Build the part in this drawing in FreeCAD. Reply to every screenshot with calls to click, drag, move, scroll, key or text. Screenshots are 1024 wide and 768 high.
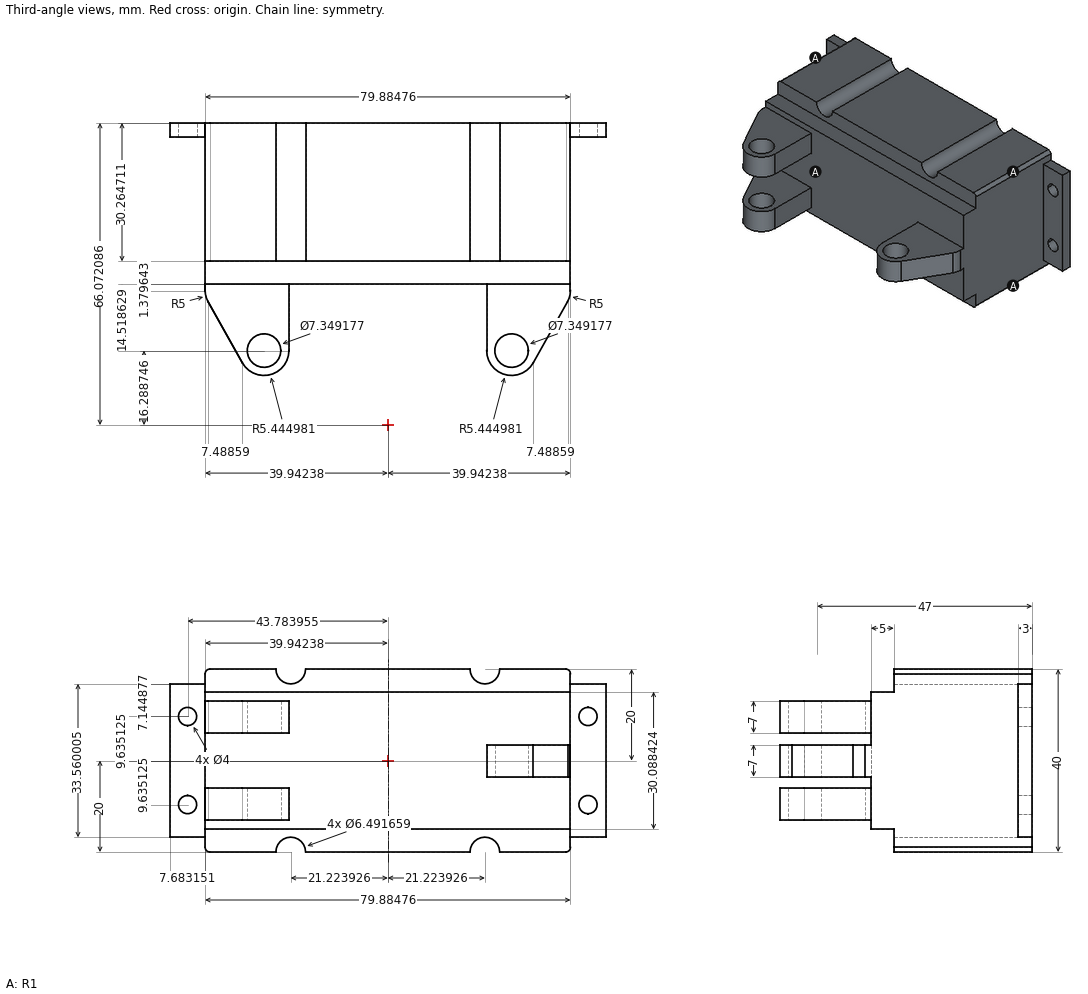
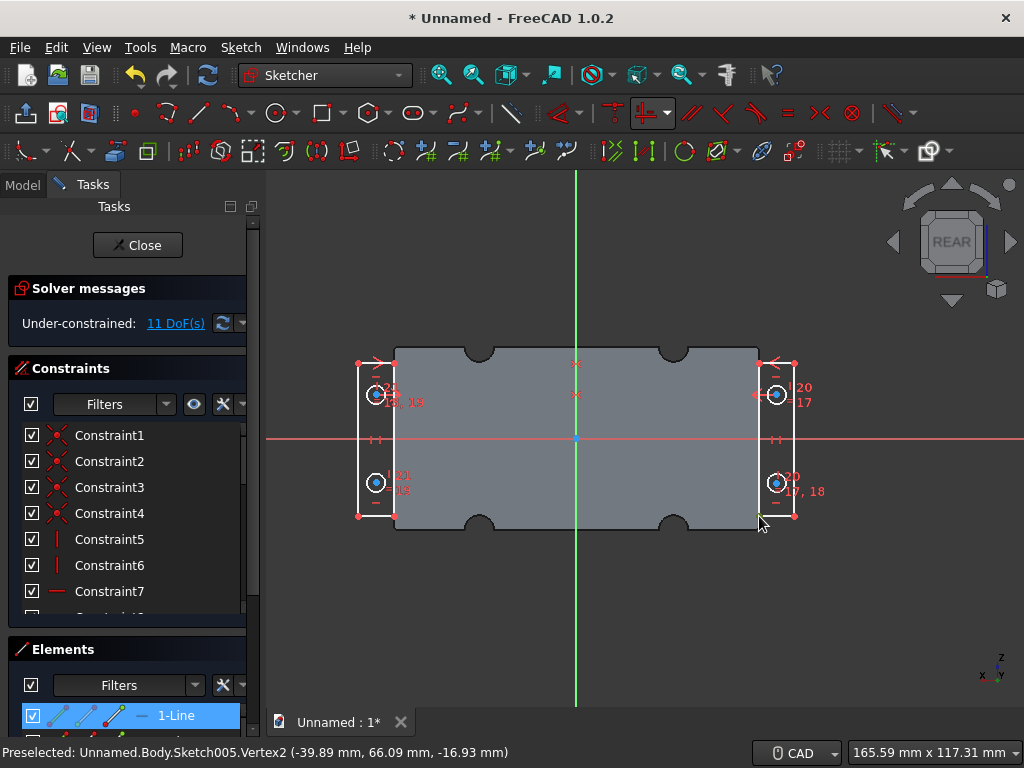
click(394, 516)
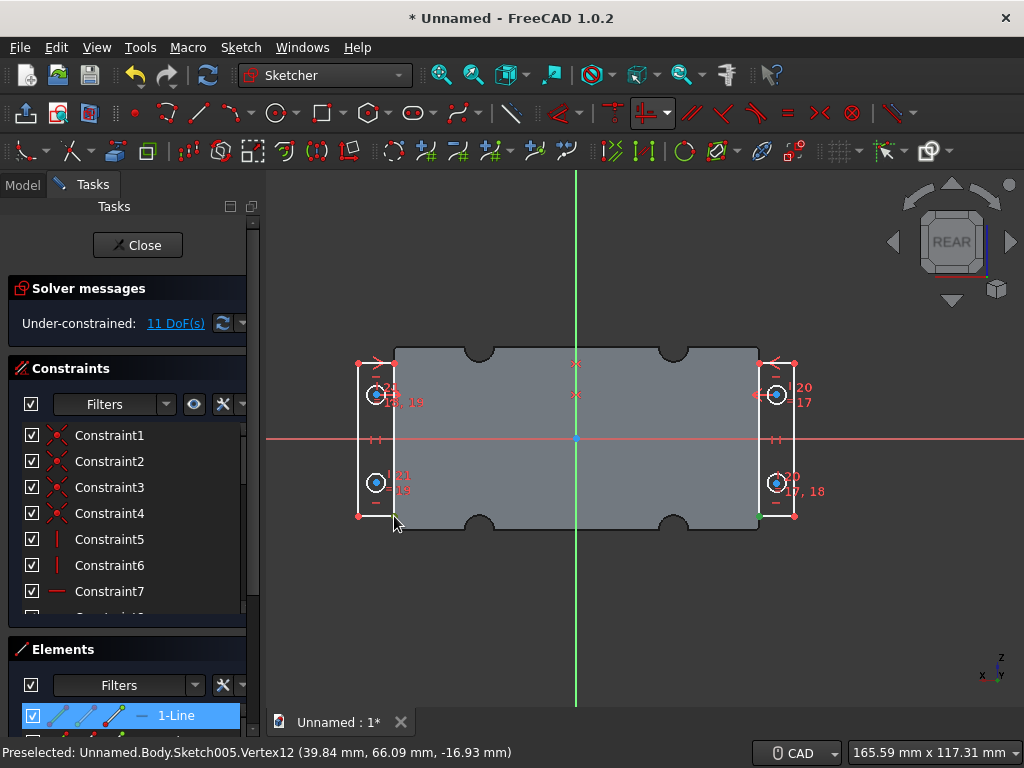
click(576, 645)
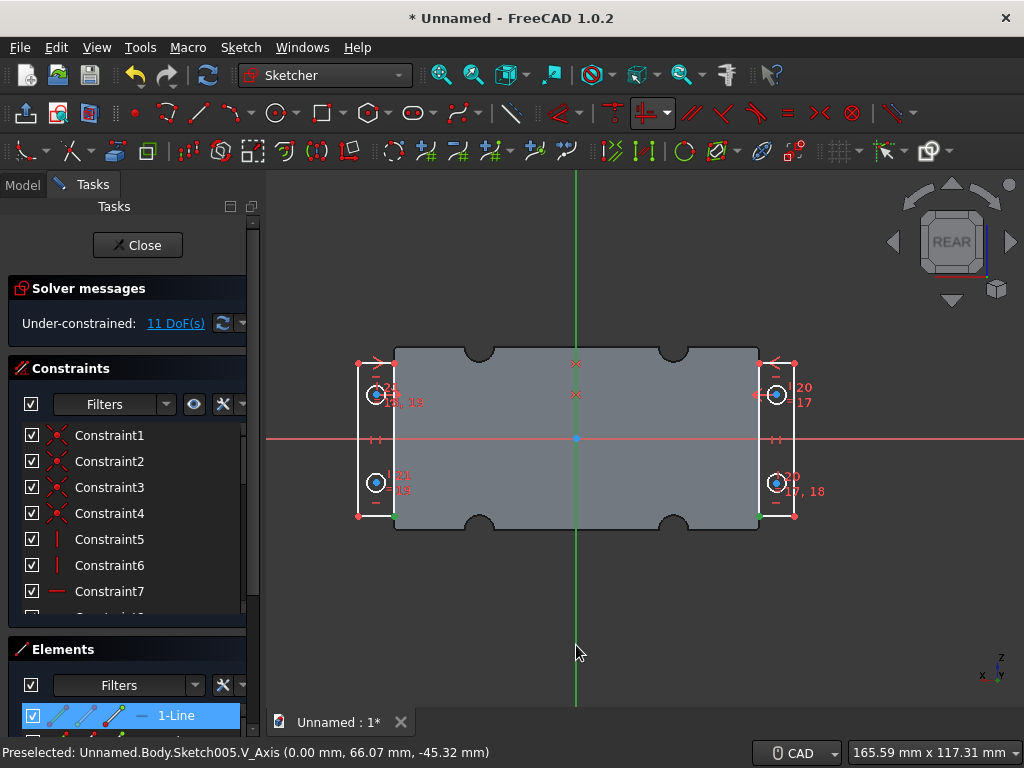
click(820, 114)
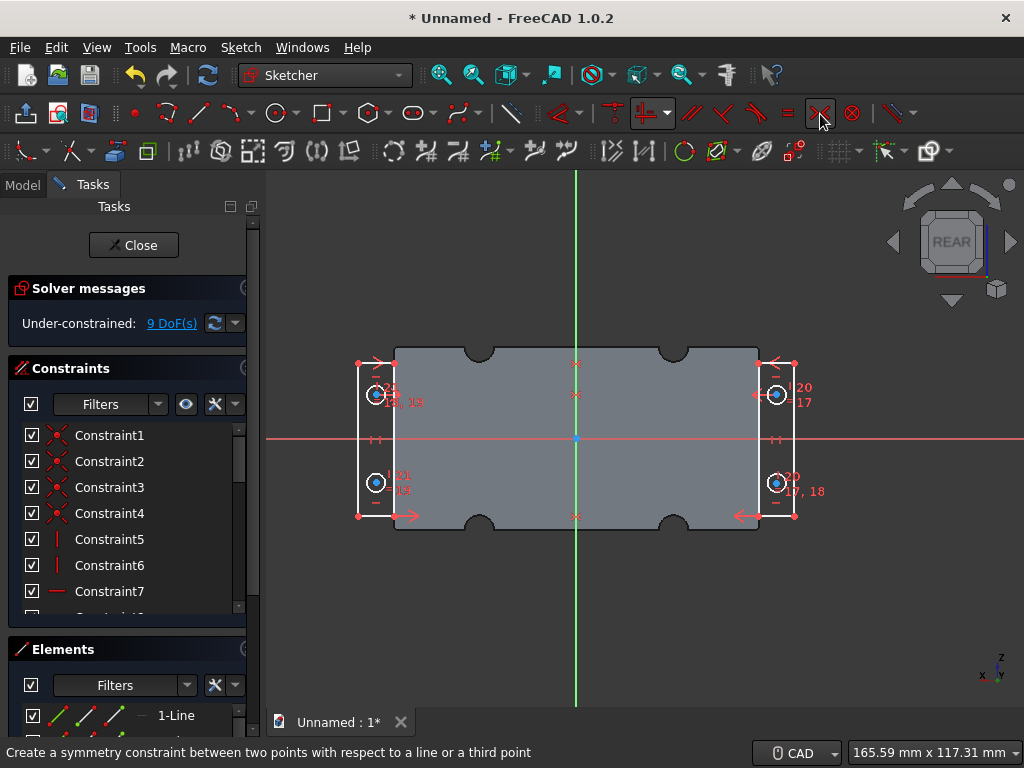
key(d)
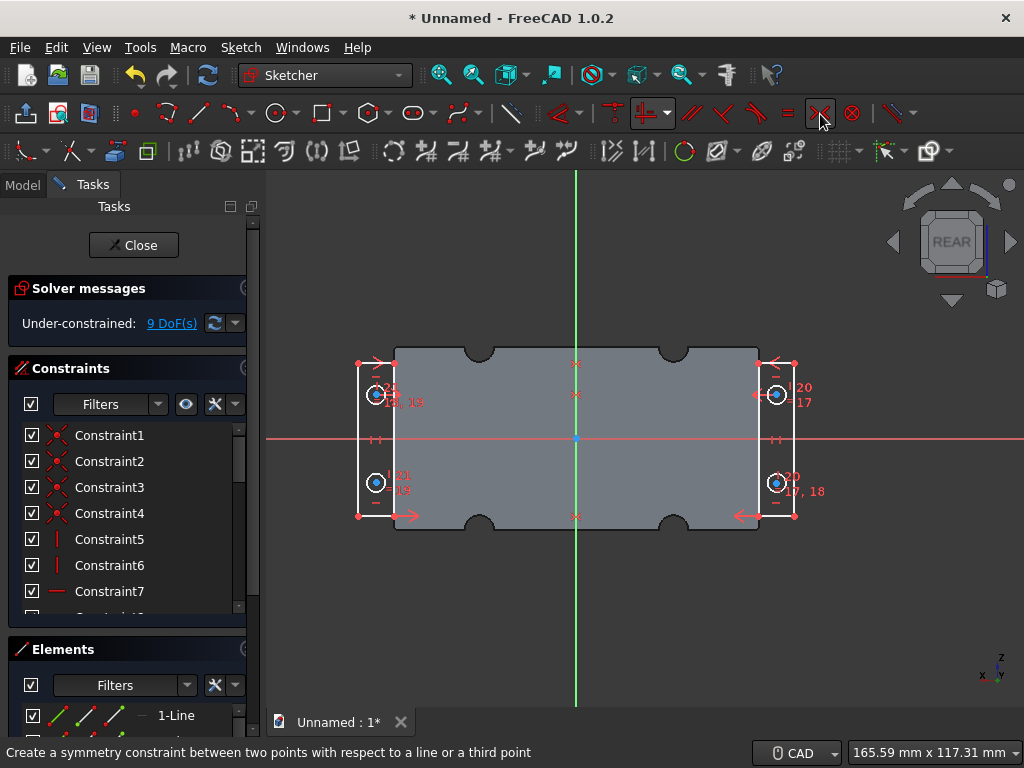
scroll(783, 388, up, 4)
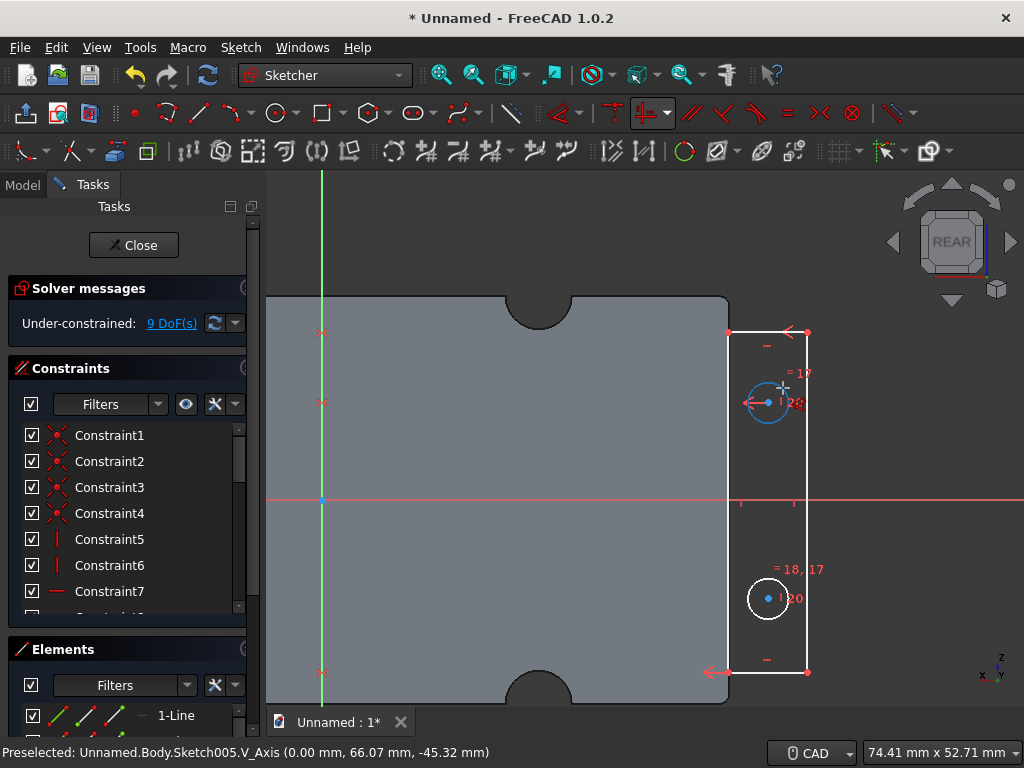
click(783, 389)
click(784, 353)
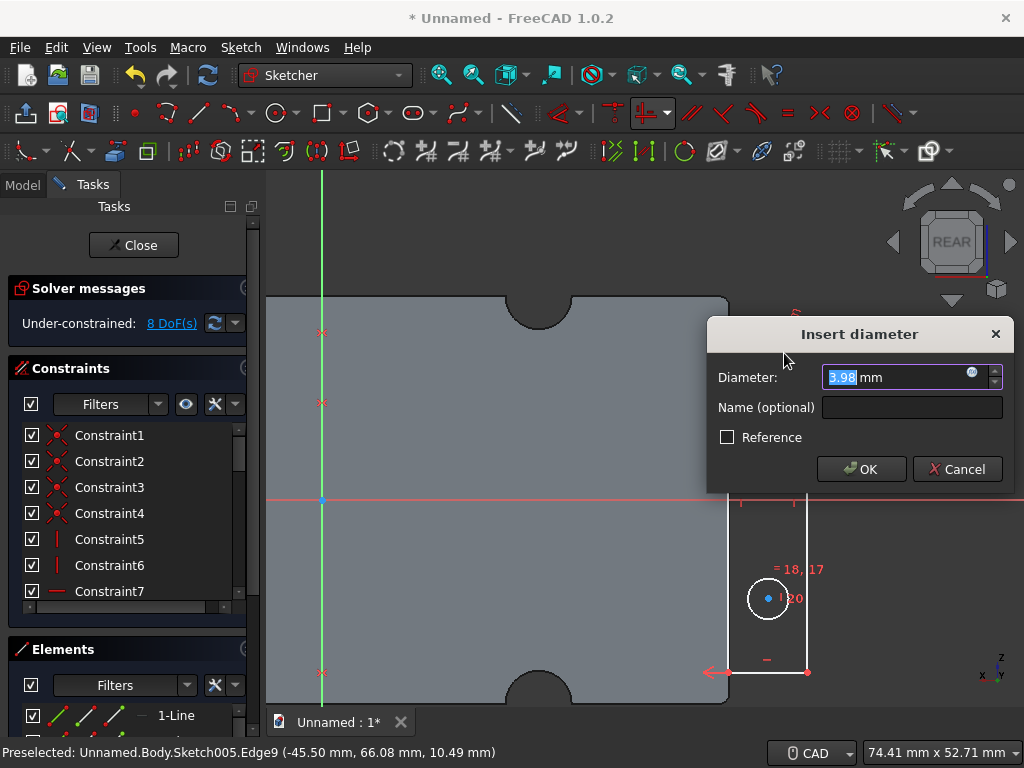
text(4)
key(Return)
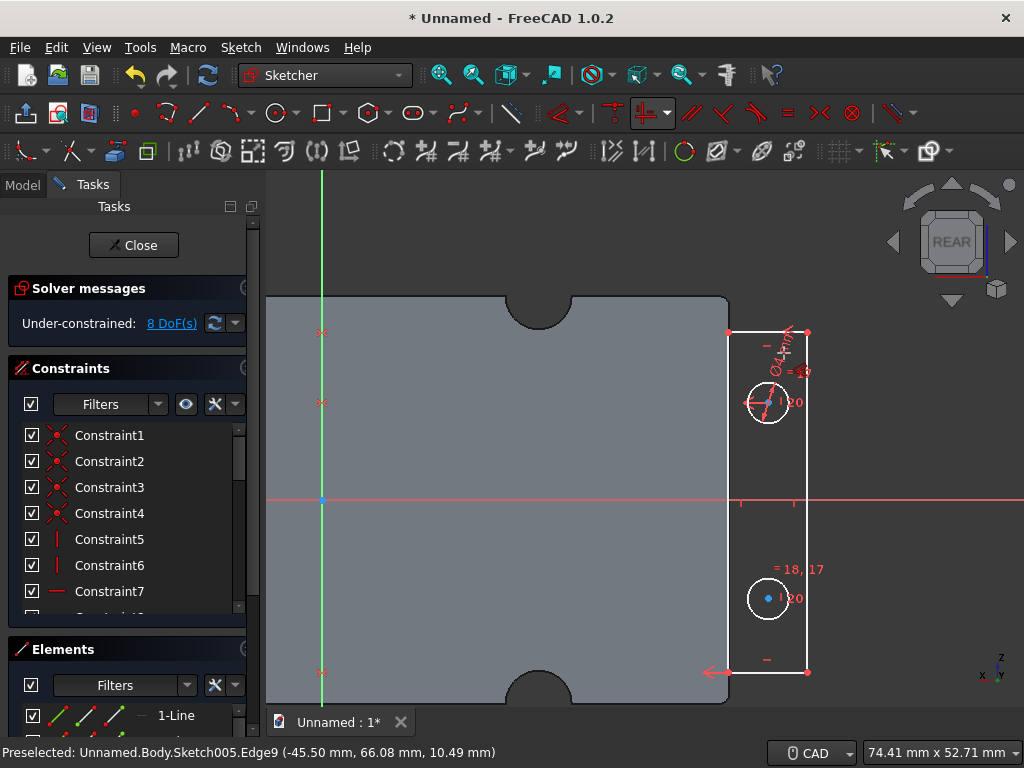
click(752, 673)
click(768, 639)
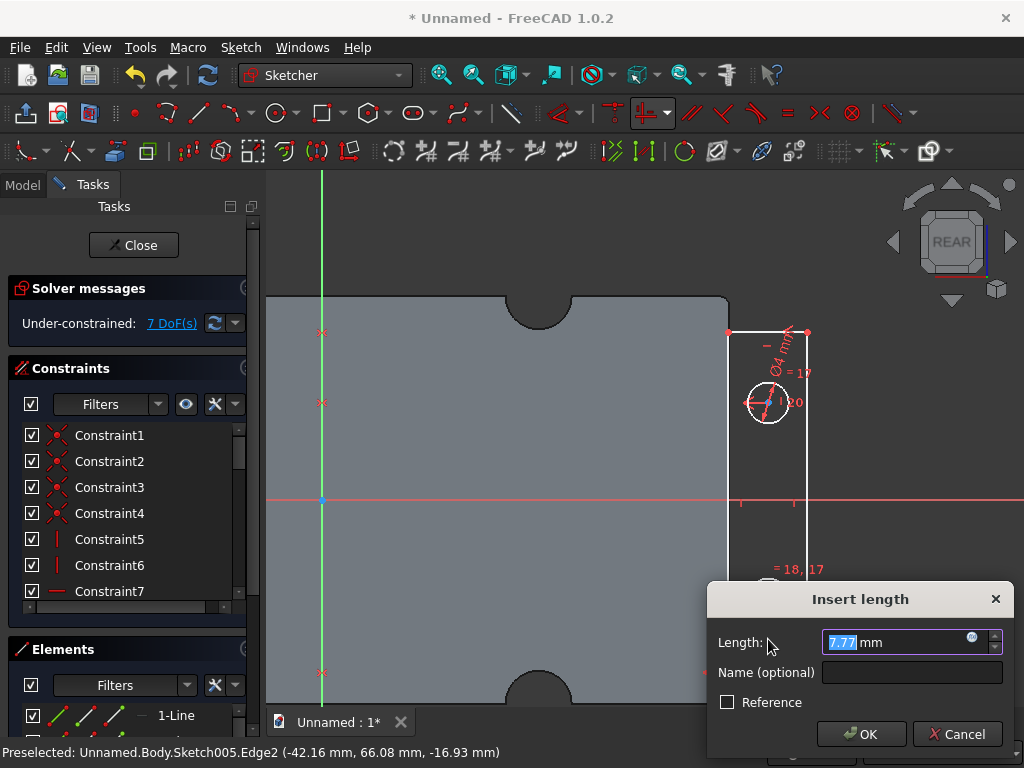
text(7.683151)
key(Return)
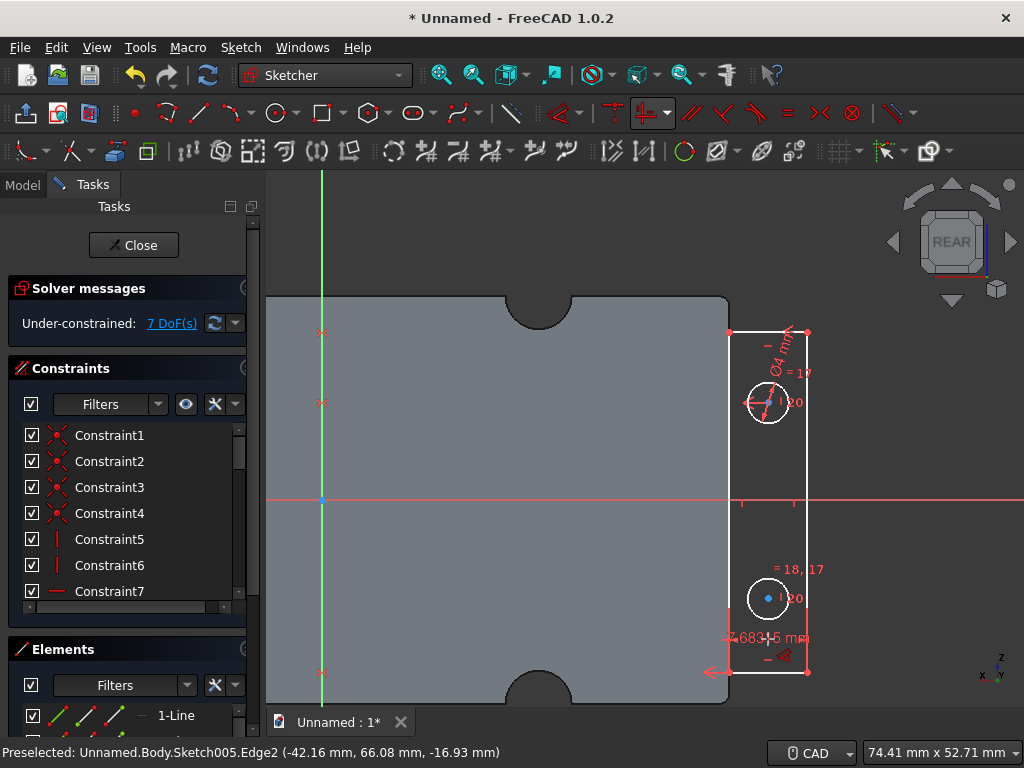
click(768, 403)
click(826, 451)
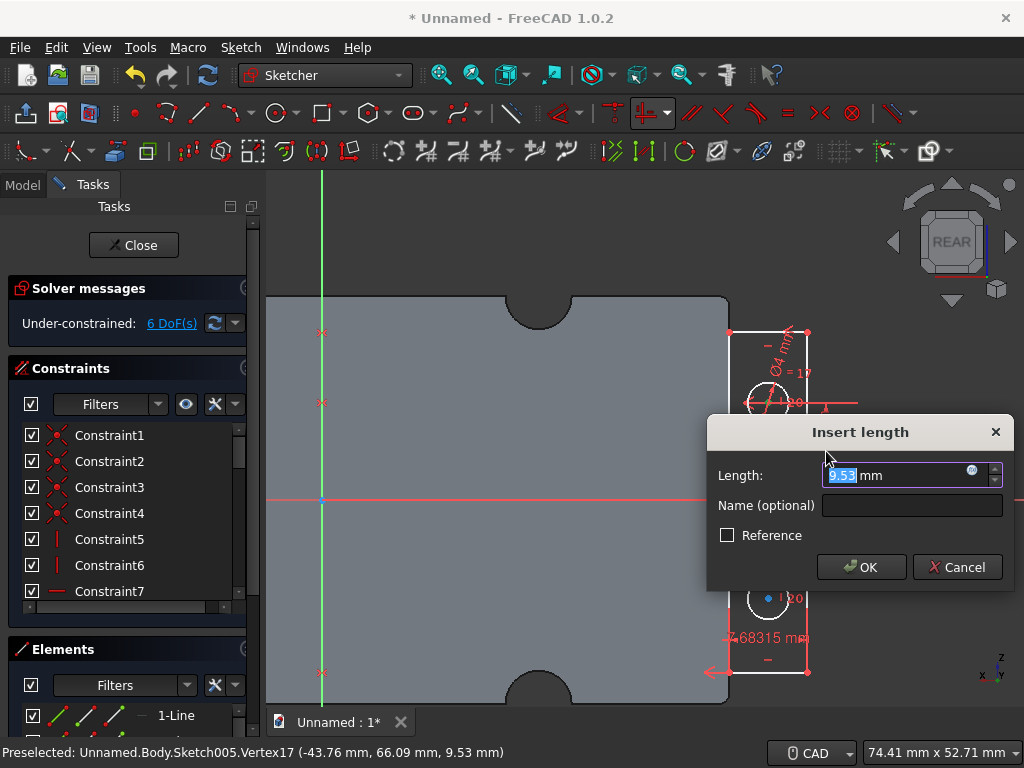
text(9.635125)
key(Return)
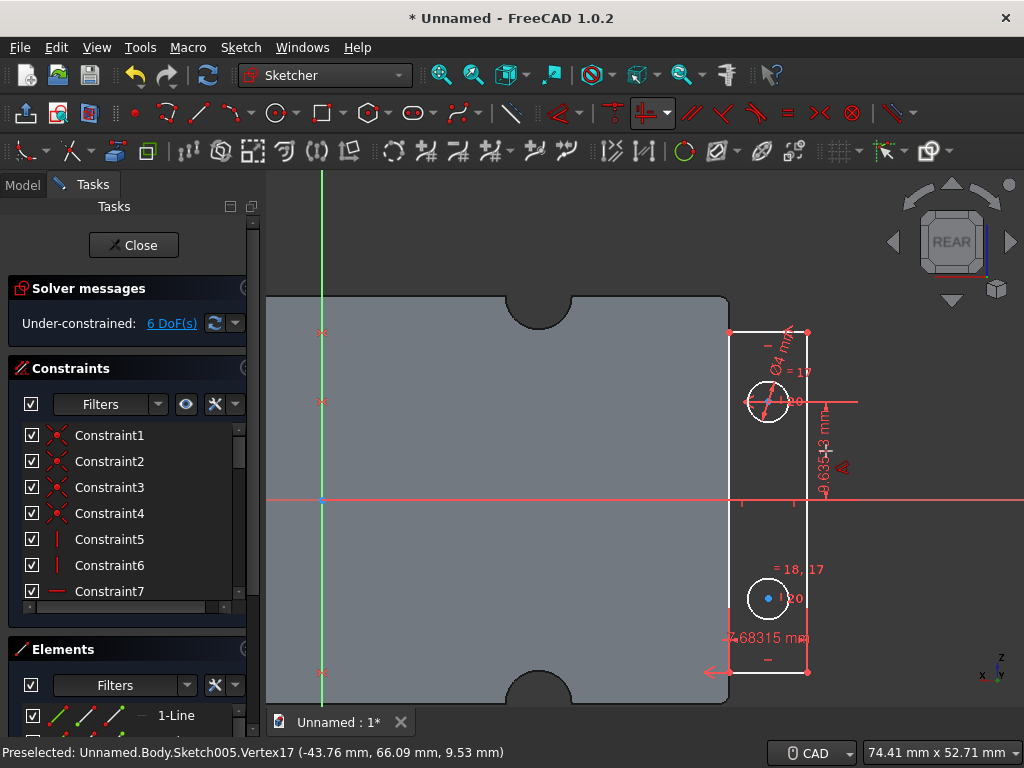
click(768, 599)
click(826, 549)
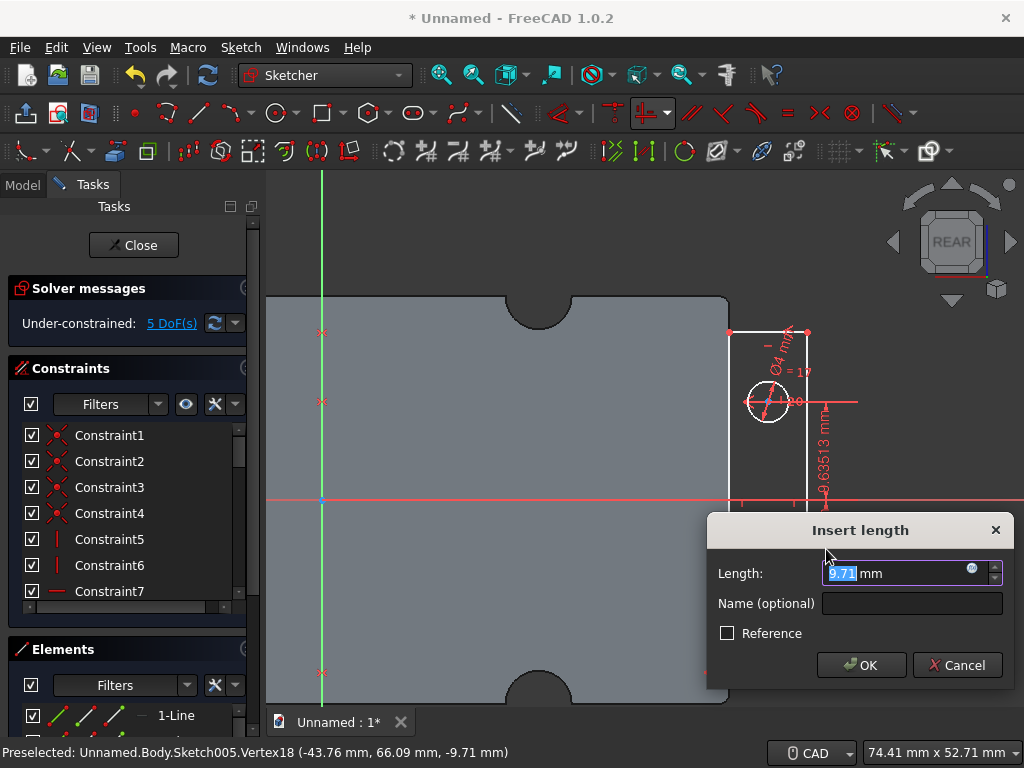
text(9.635125)
key(Return)